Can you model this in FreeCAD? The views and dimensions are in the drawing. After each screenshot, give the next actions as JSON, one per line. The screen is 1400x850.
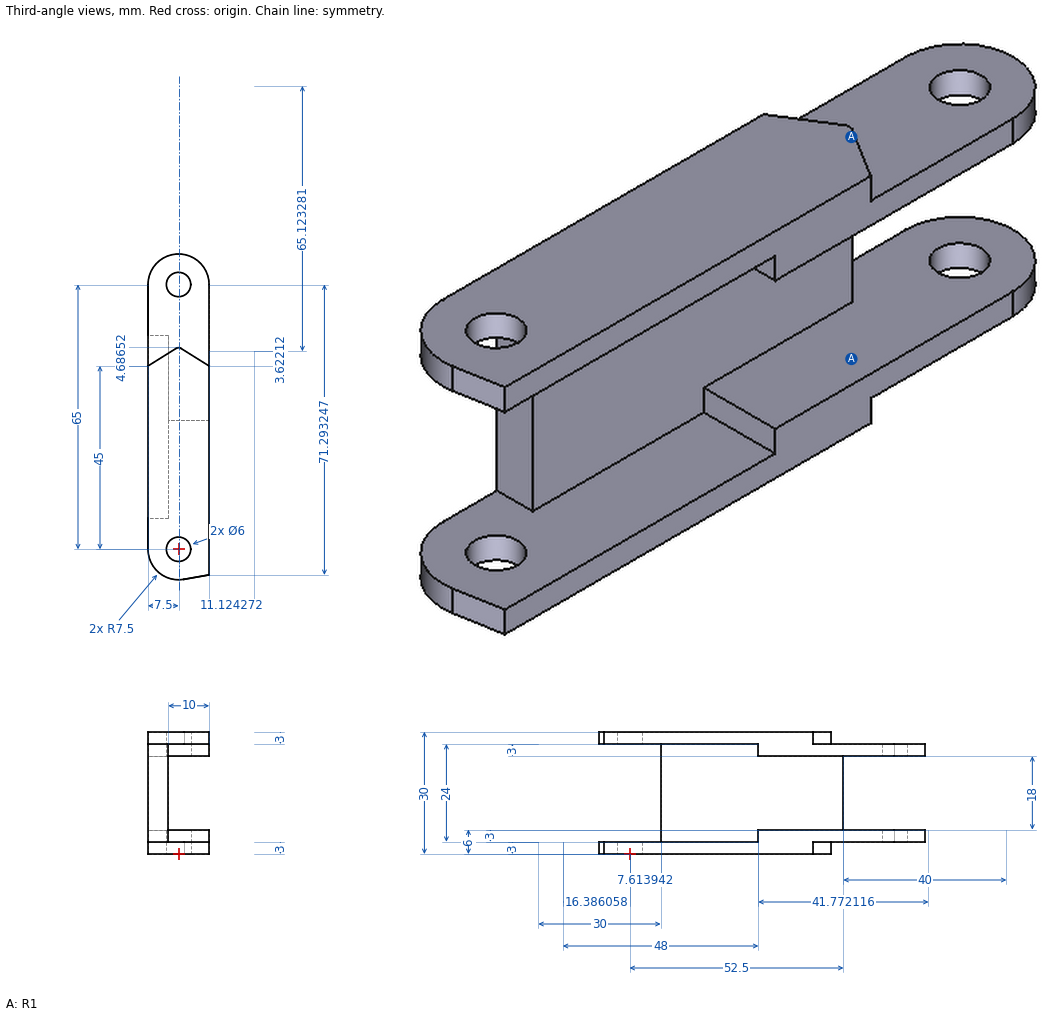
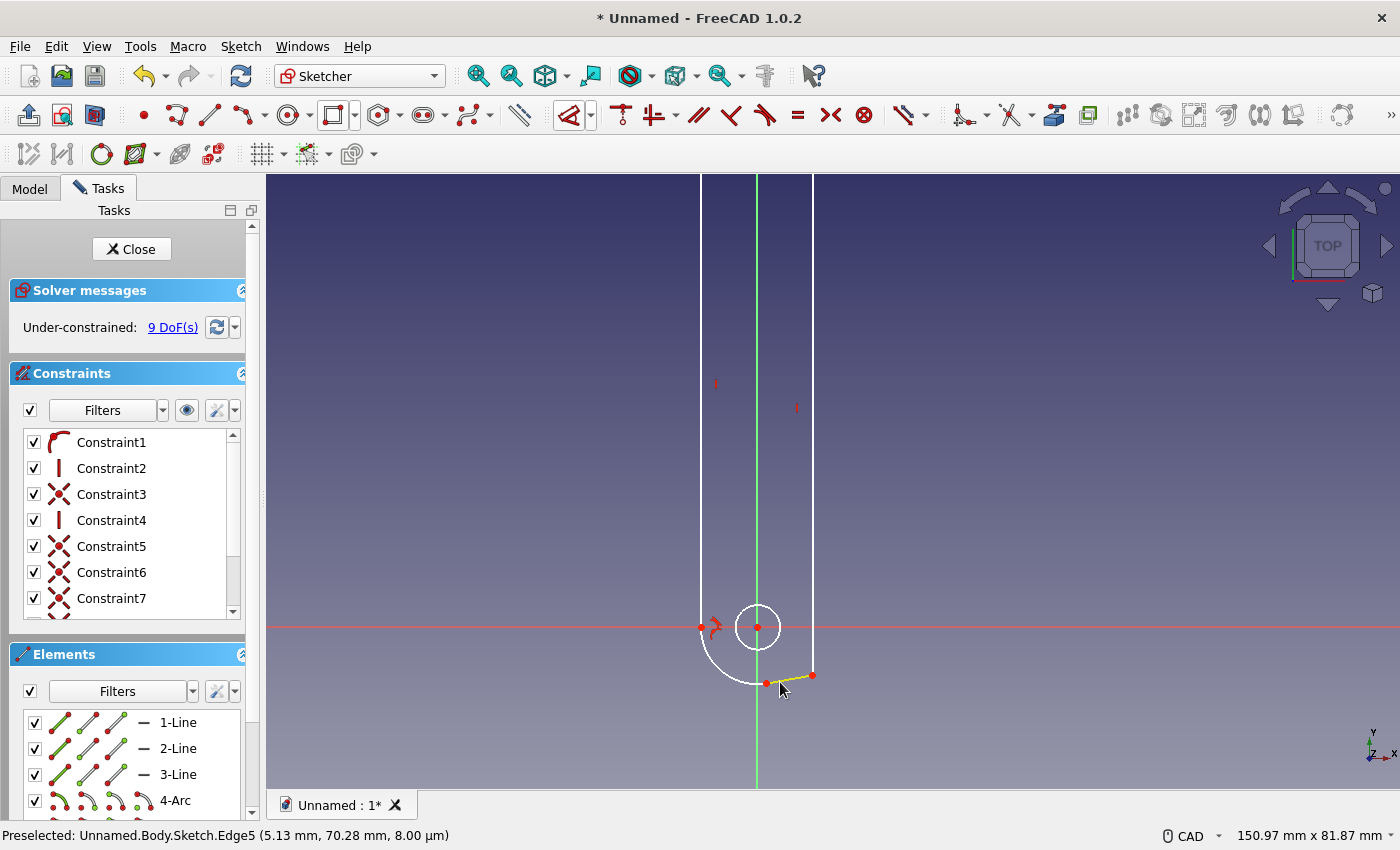
{"action": "left_click", "coordinate": [780, 681]}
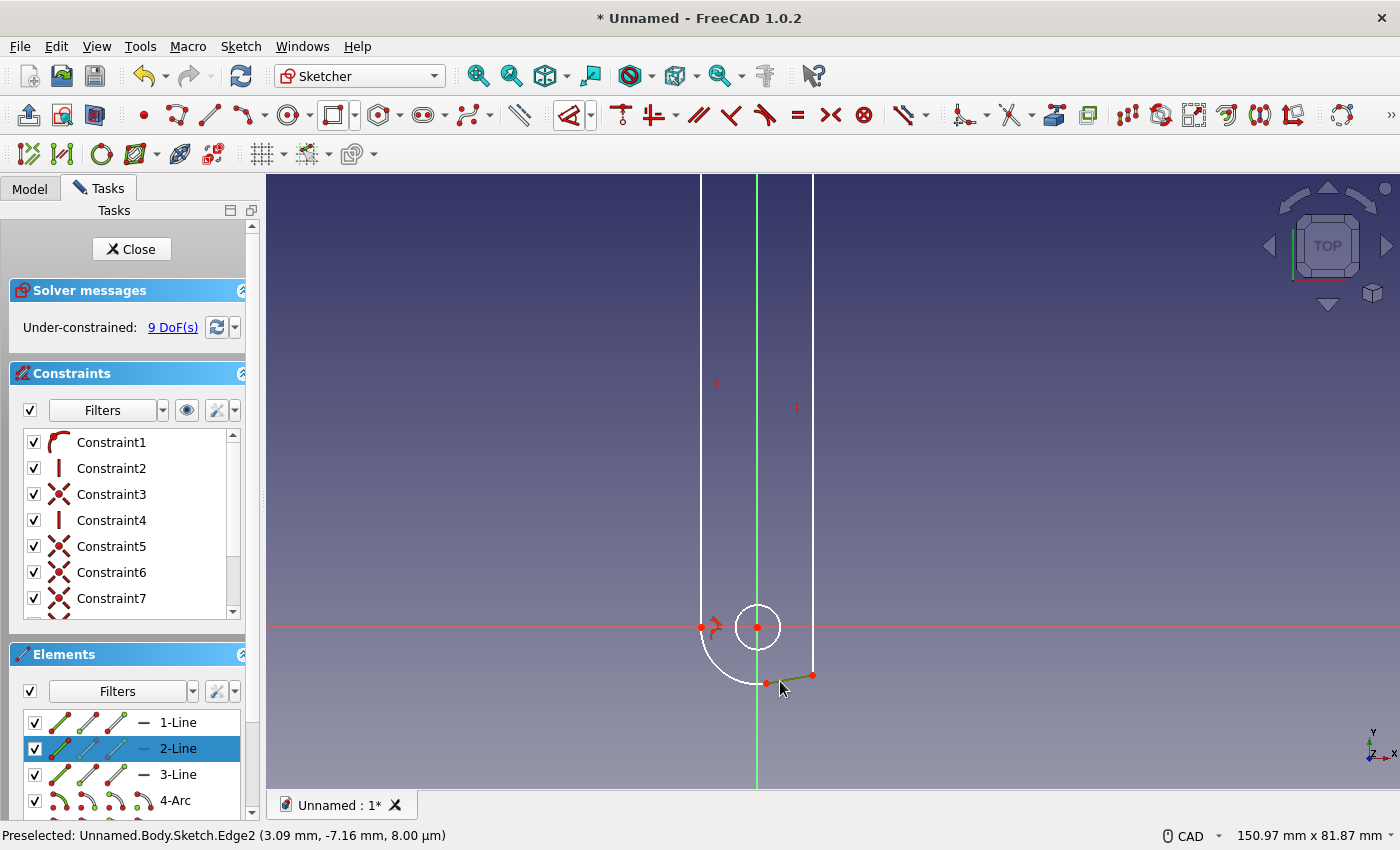
{"action": "left_click", "coordinate": [708, 656]}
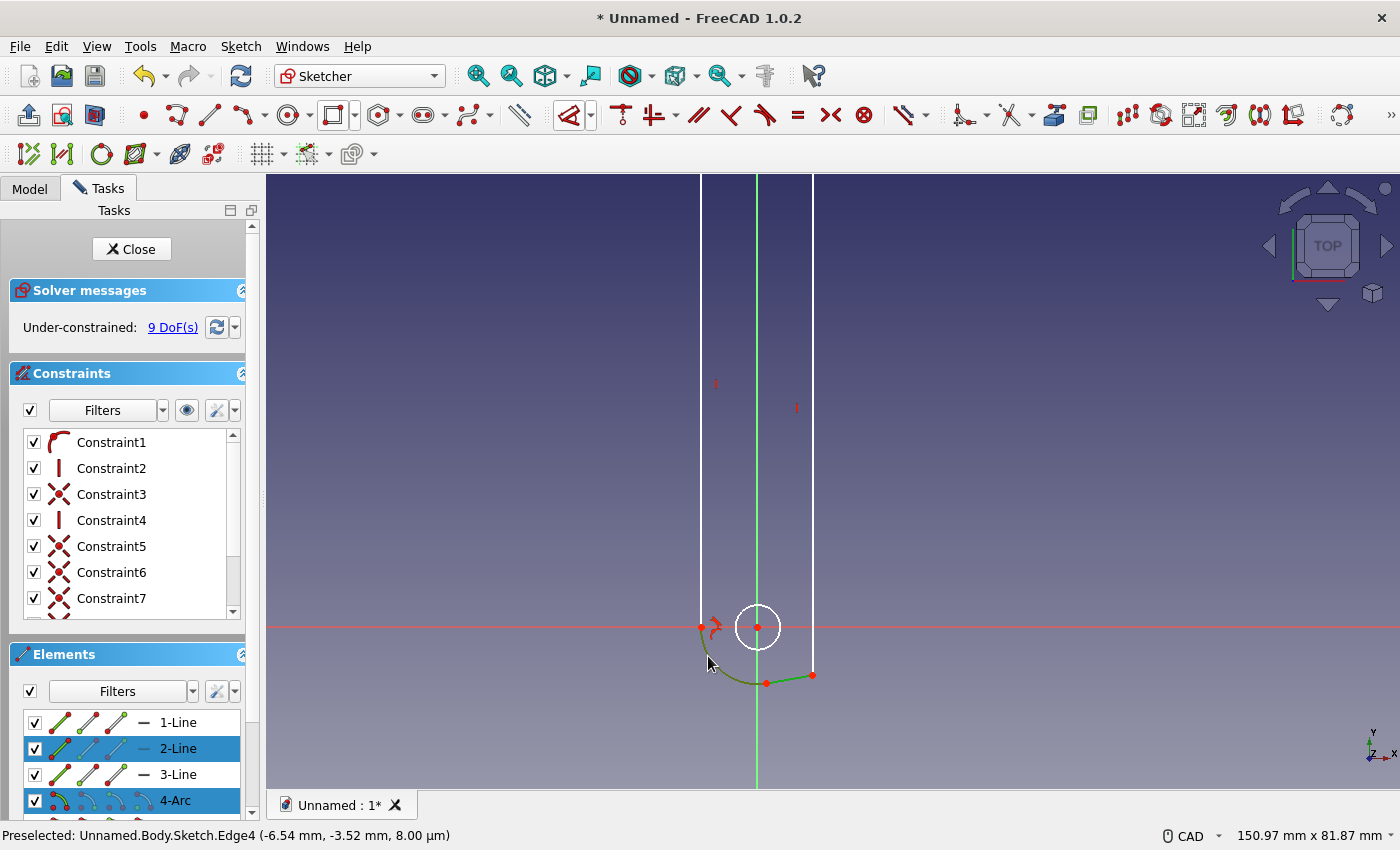
{"action": "key", "text": "t"}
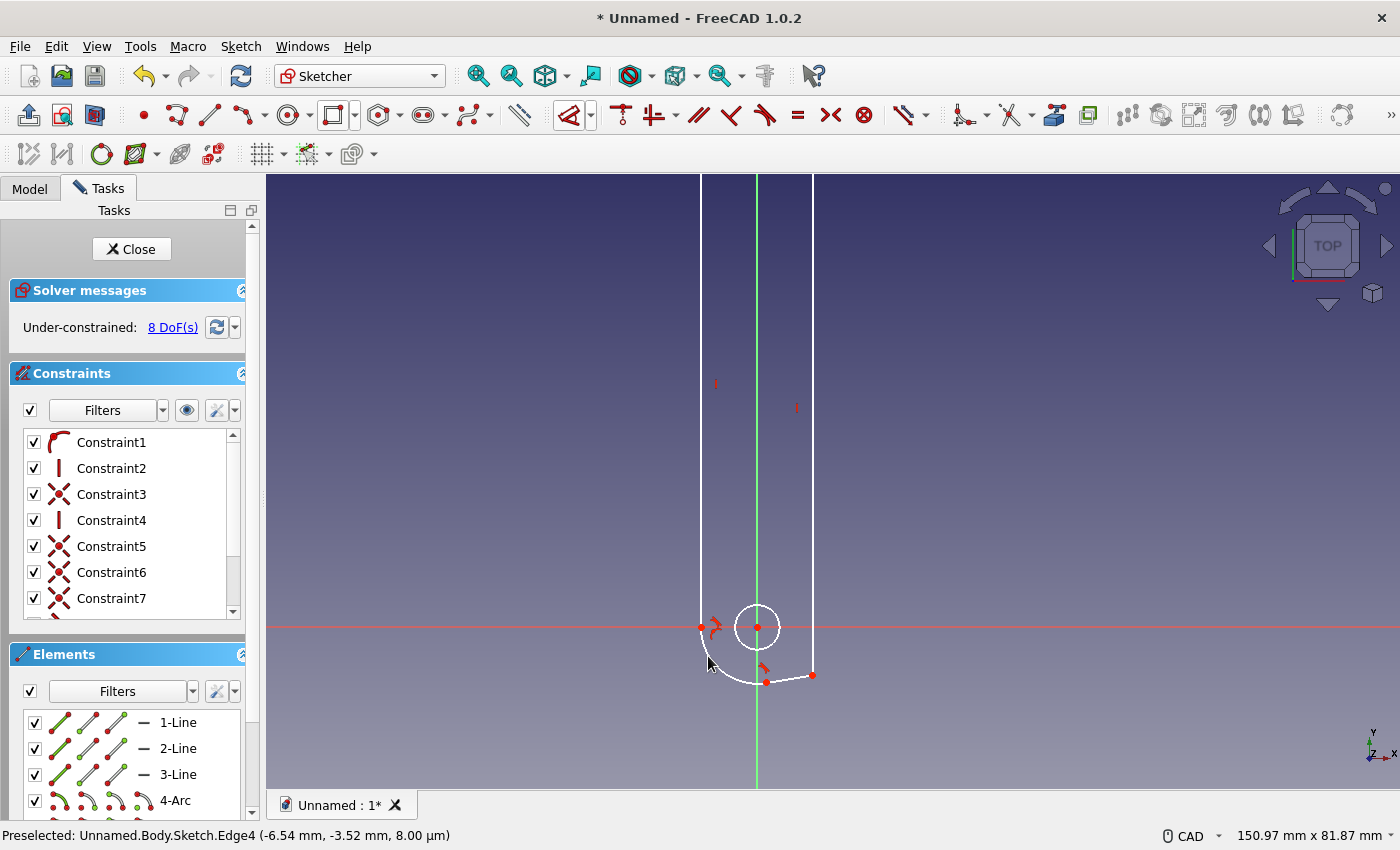
{"action": "left_click", "coordinate": [813, 515]}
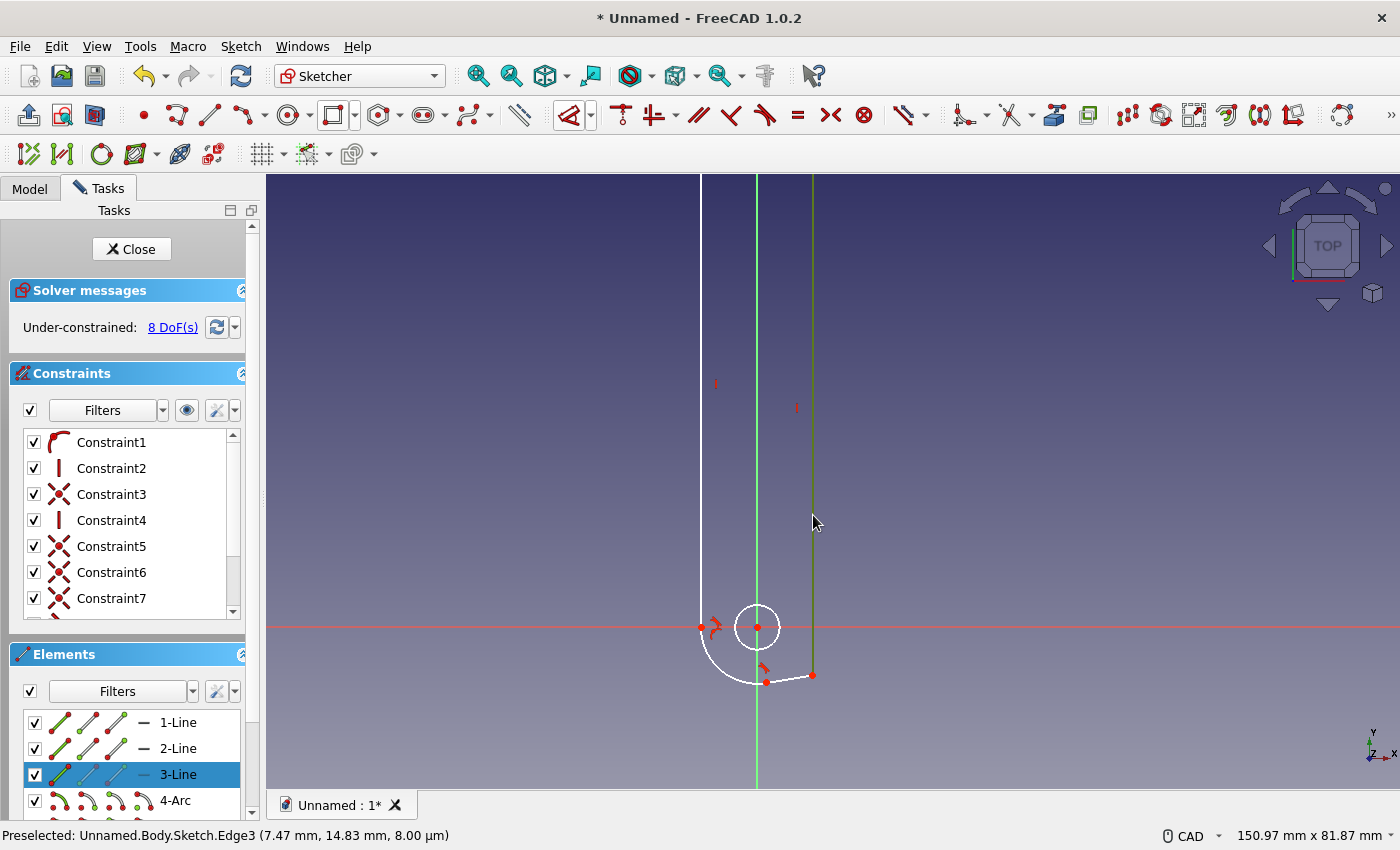
{"action": "scroll", "coordinate": [780, 682], "scroll_direction": "down", "scroll_amount": 2}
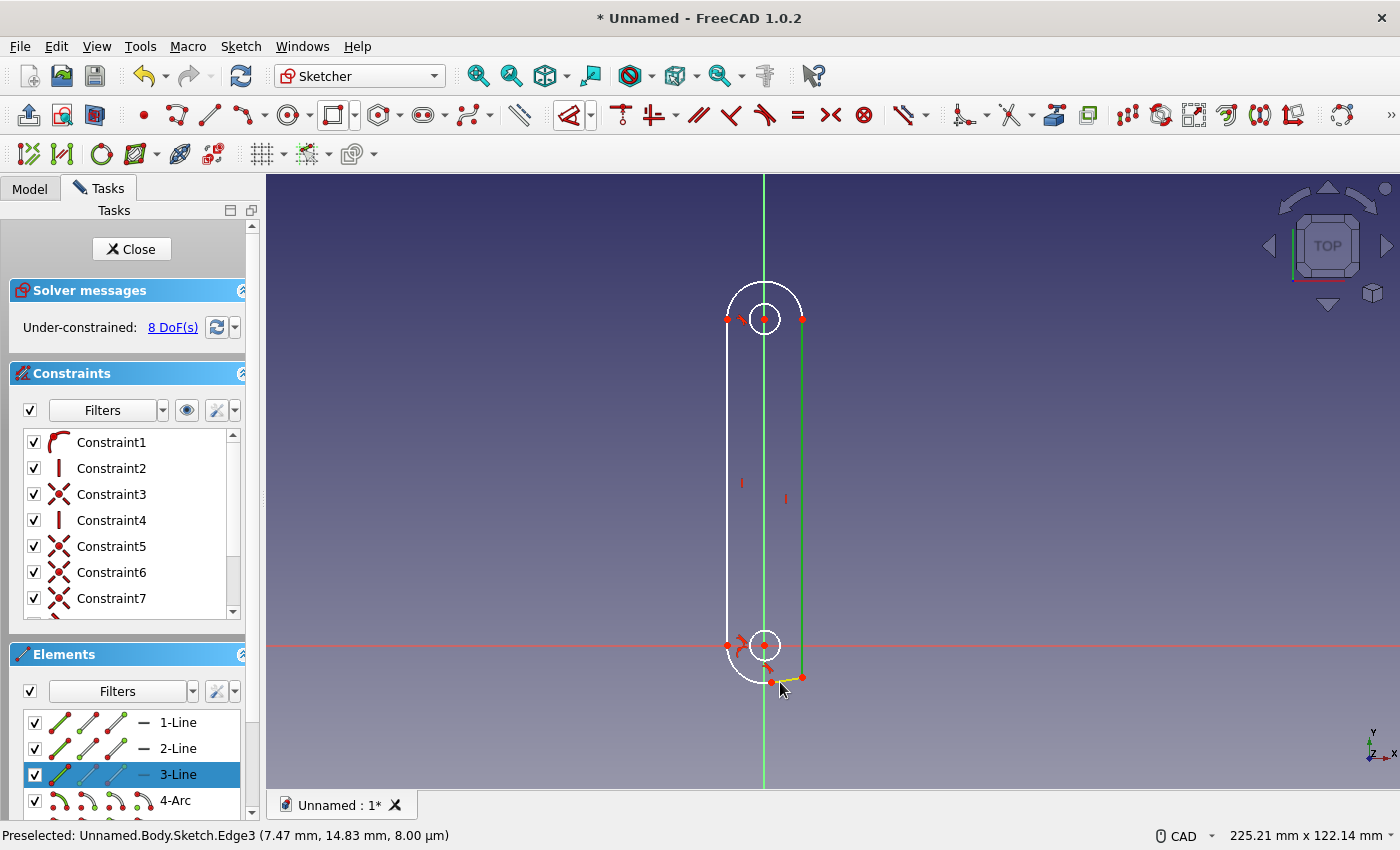
{"action": "left_click", "coordinate": [787, 289]}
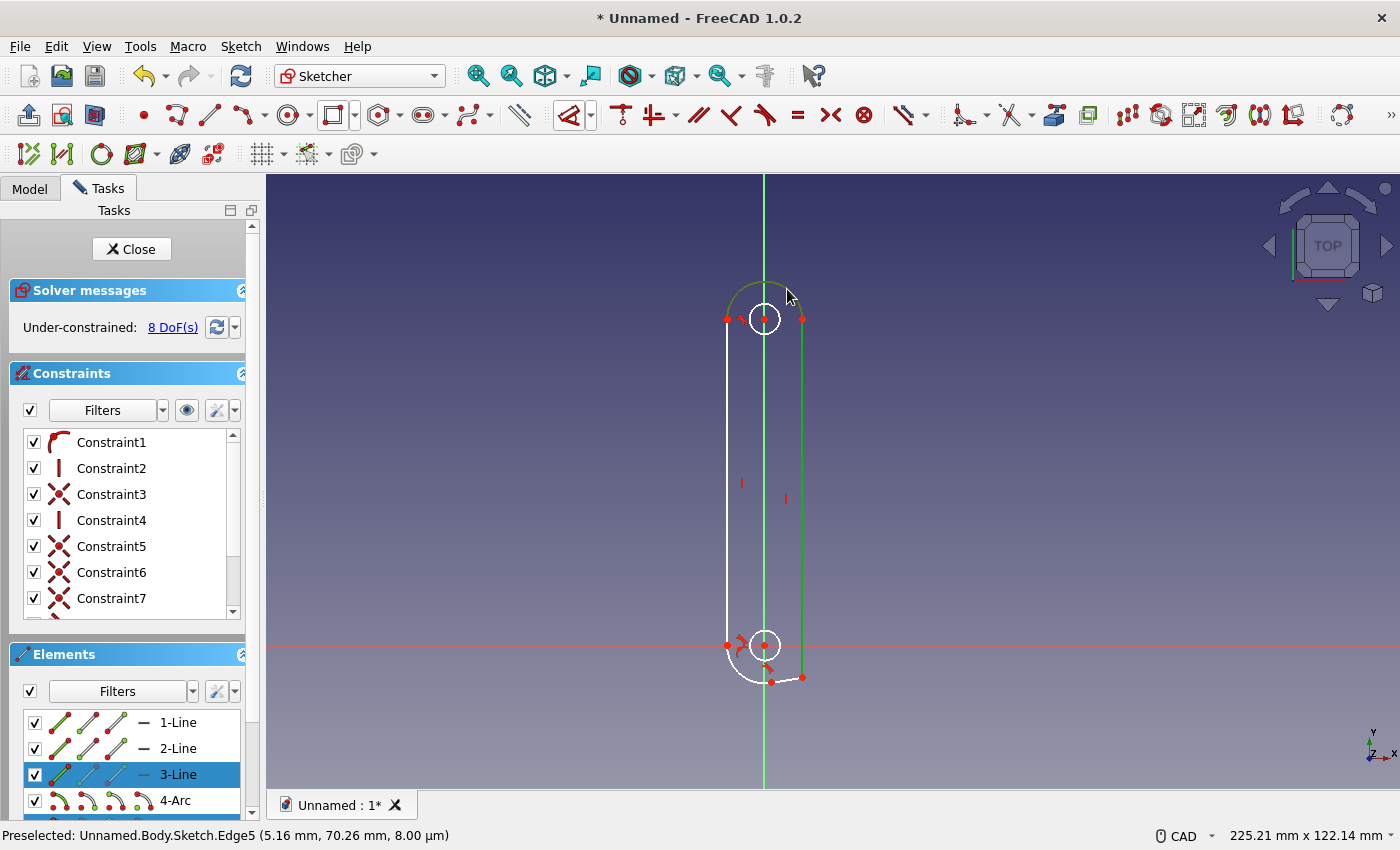
{"action": "key", "text": "t"}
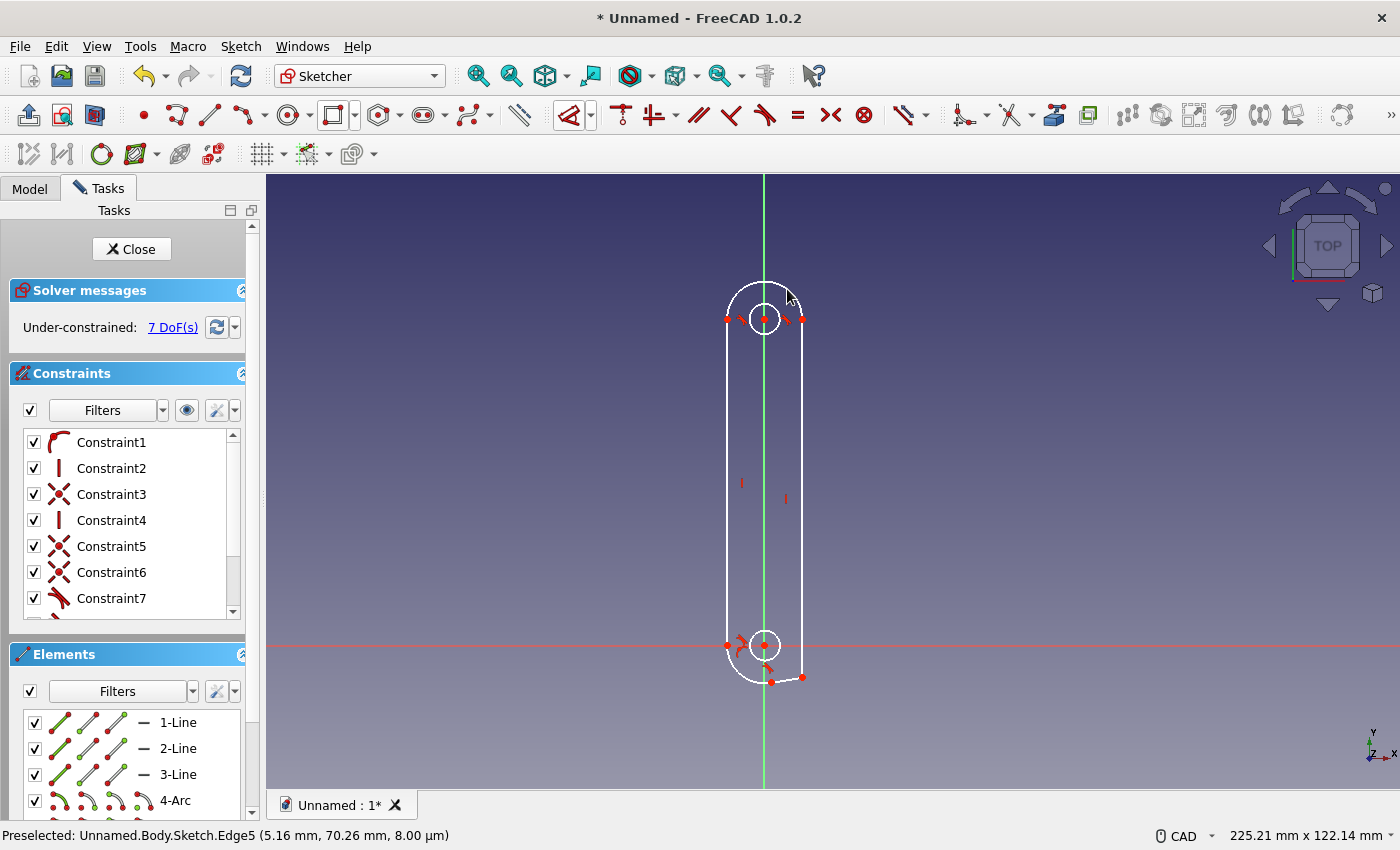
{"action": "left_click", "coordinate": [732, 664]}